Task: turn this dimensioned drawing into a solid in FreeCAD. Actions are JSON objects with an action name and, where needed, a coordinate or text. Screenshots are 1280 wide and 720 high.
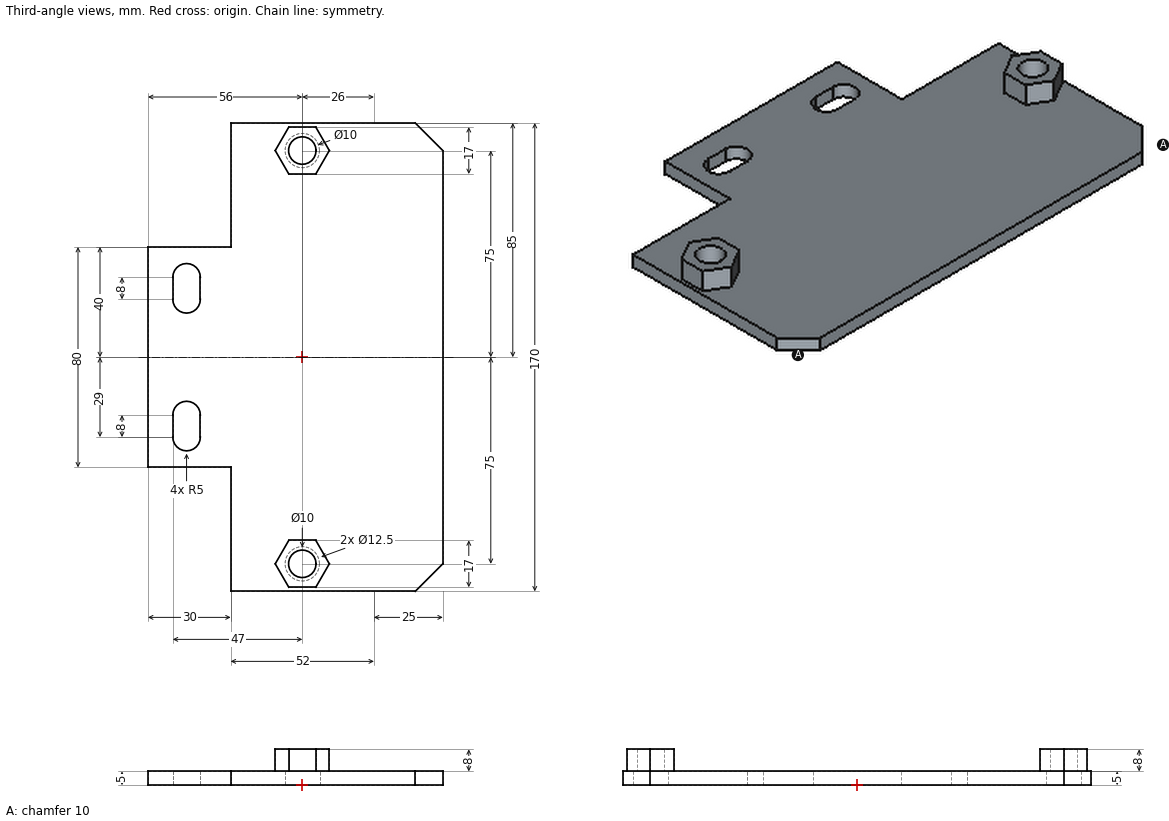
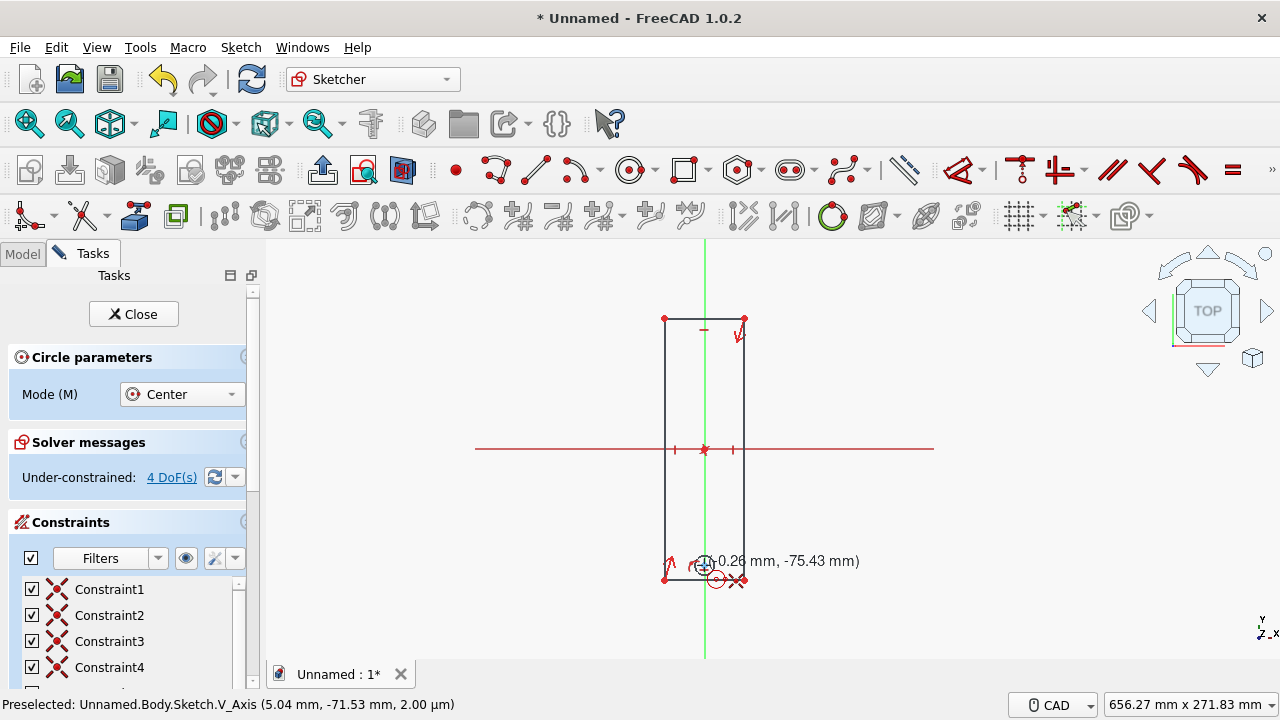
{"action": "scroll", "coordinate": [705, 333], "scroll_direction": "up", "scroll_amount": 5}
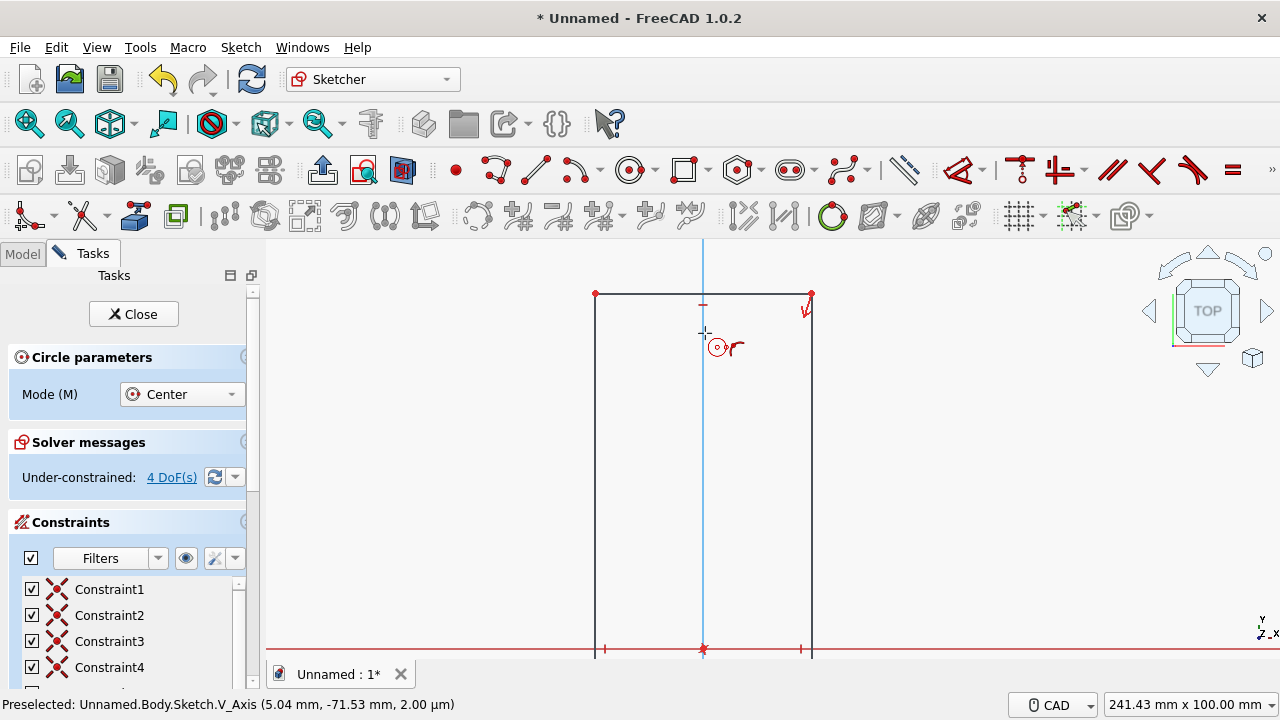
{"action": "left_click", "coordinate": [703, 334]}
{"action": "left_click", "coordinate": [722, 315]}
{"action": "key", "text": "Escape"}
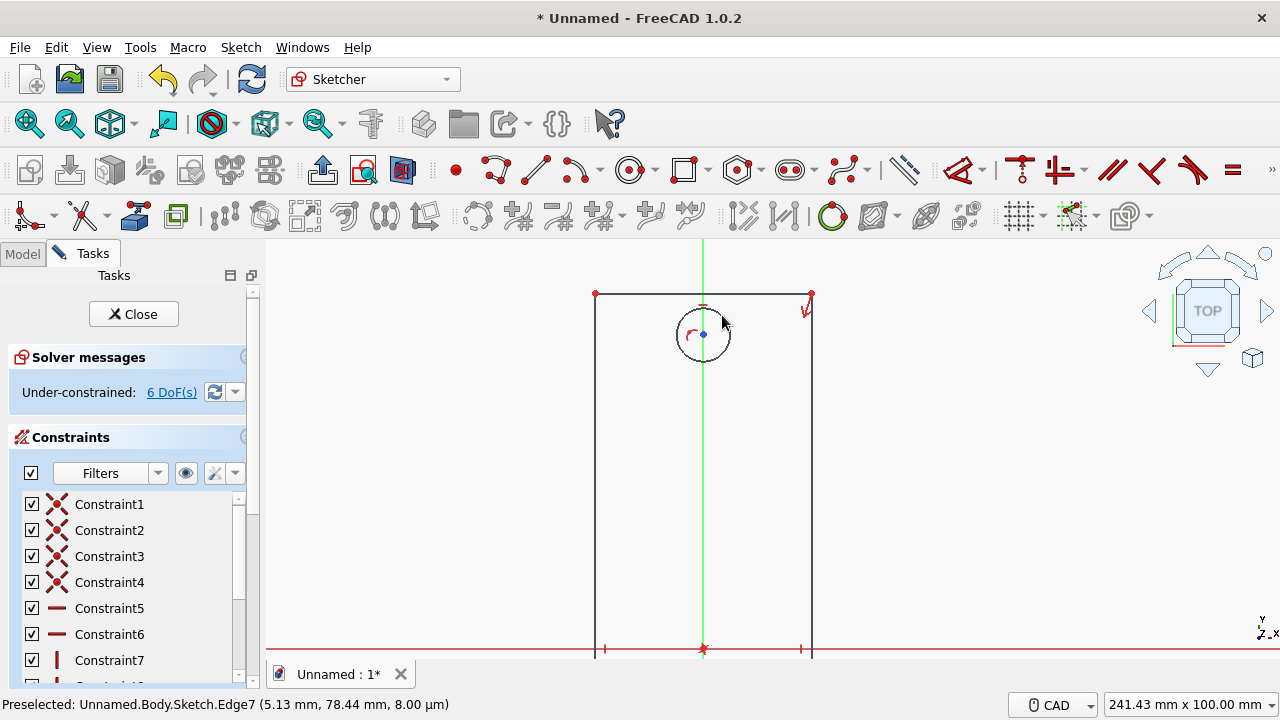
{"action": "scroll", "coordinate": [705, 333], "scroll_direction": "down", "scroll_amount": 5}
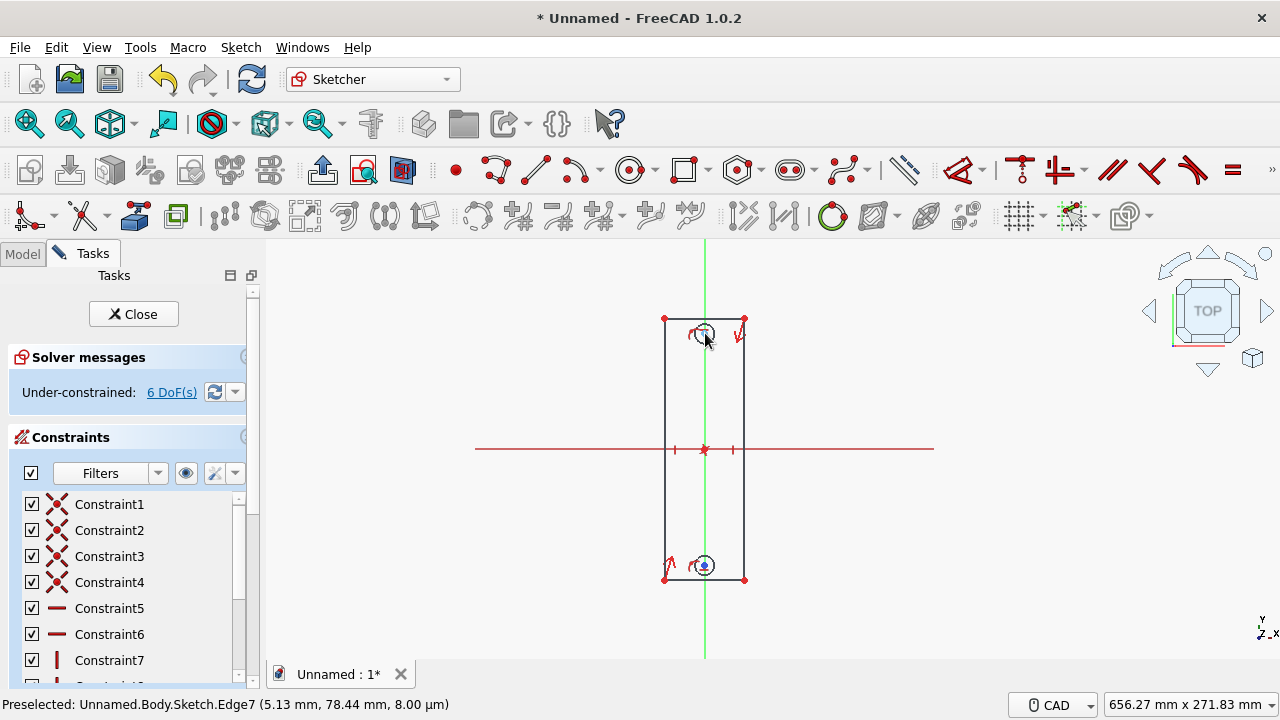
{"action": "scroll", "coordinate": [711, 559], "scroll_direction": "up", "scroll_amount": 4}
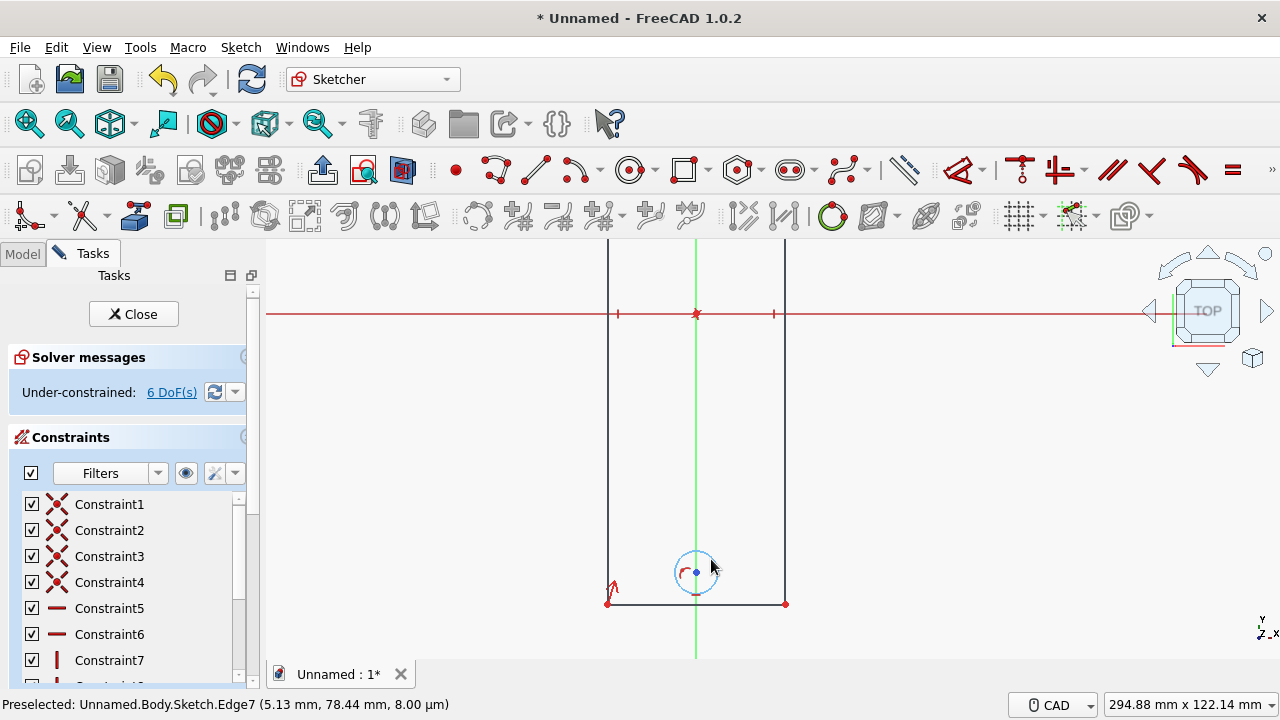
{"action": "left_click", "coordinate": [711, 557]}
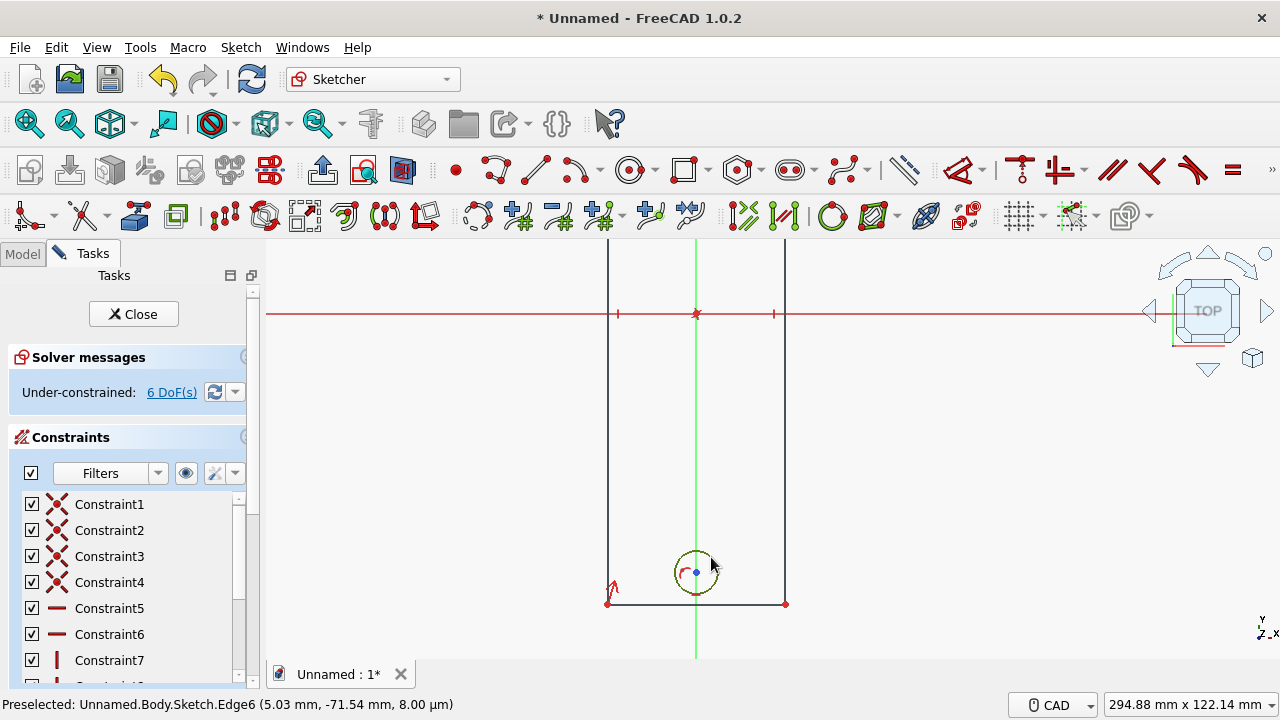
{"action": "scroll", "coordinate": [711, 559], "scroll_direction": "down", "scroll_amount": 4}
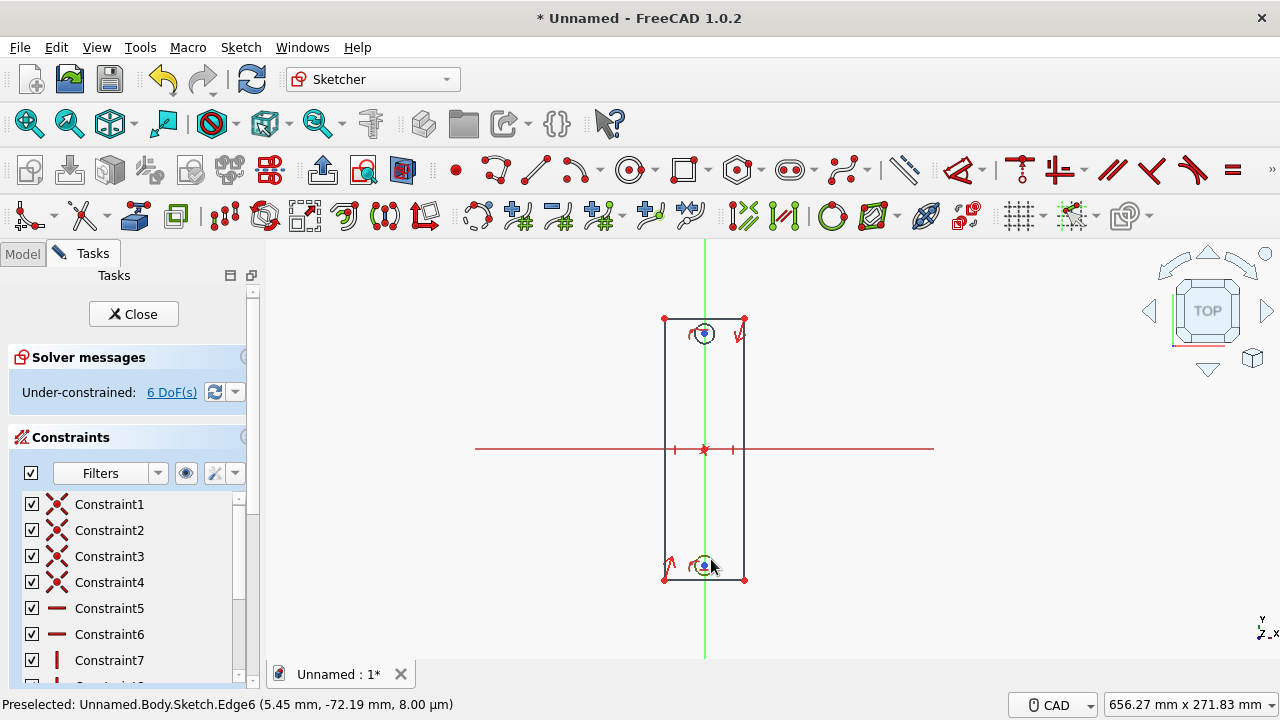
{"action": "scroll", "coordinate": [712, 327], "scroll_direction": "up", "scroll_amount": 4}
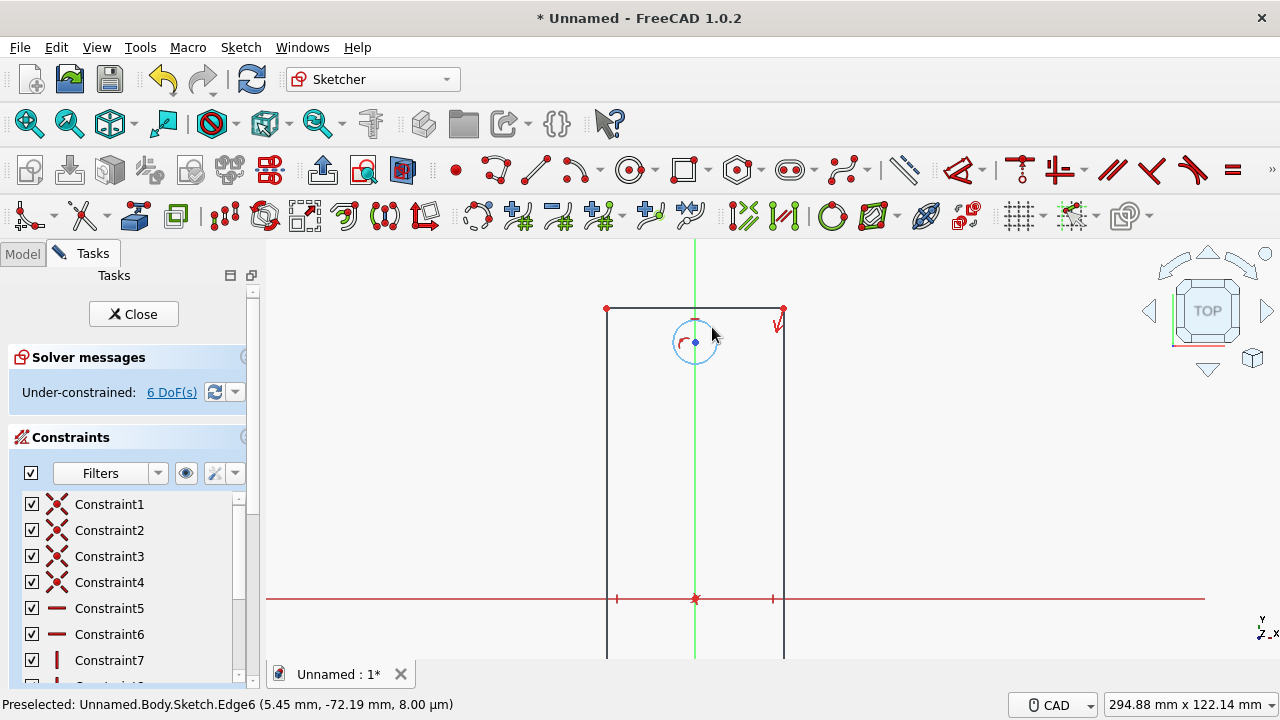
{"action": "left_click", "coordinate": [711, 327]}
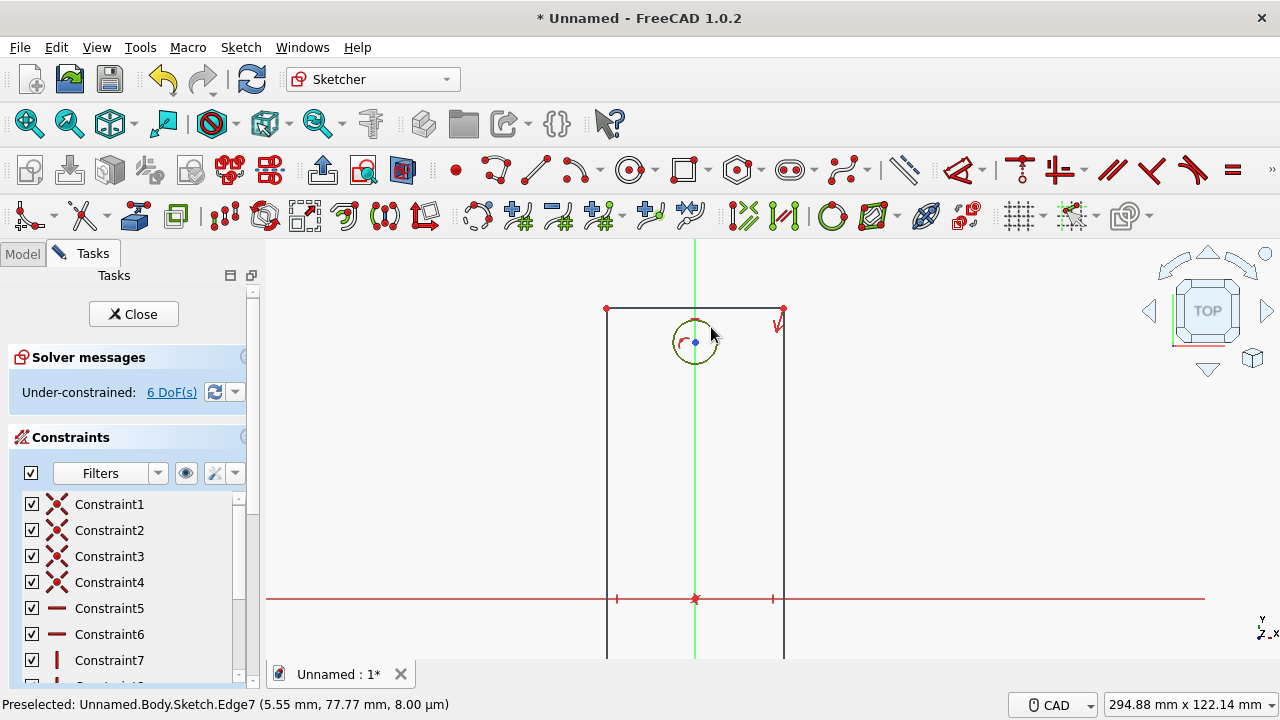
{"action": "left_click", "coordinate": [1234, 170]}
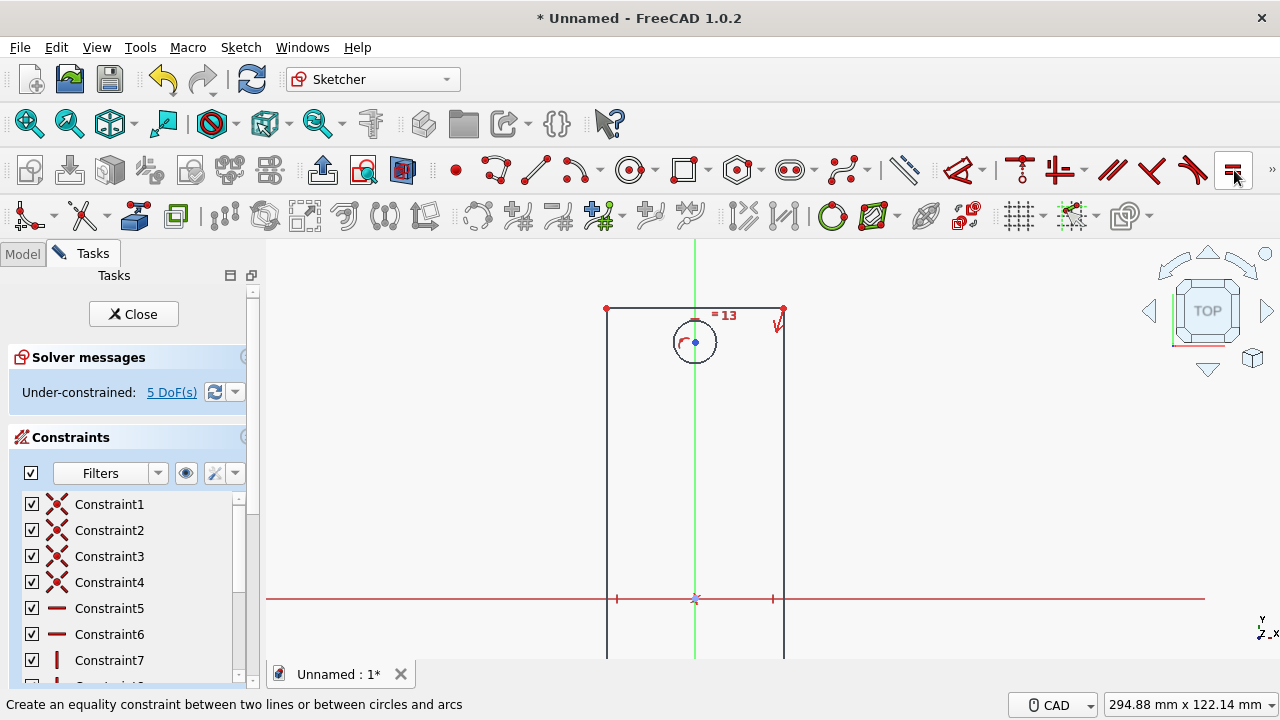
{"action": "left_click", "coordinate": [958, 170]}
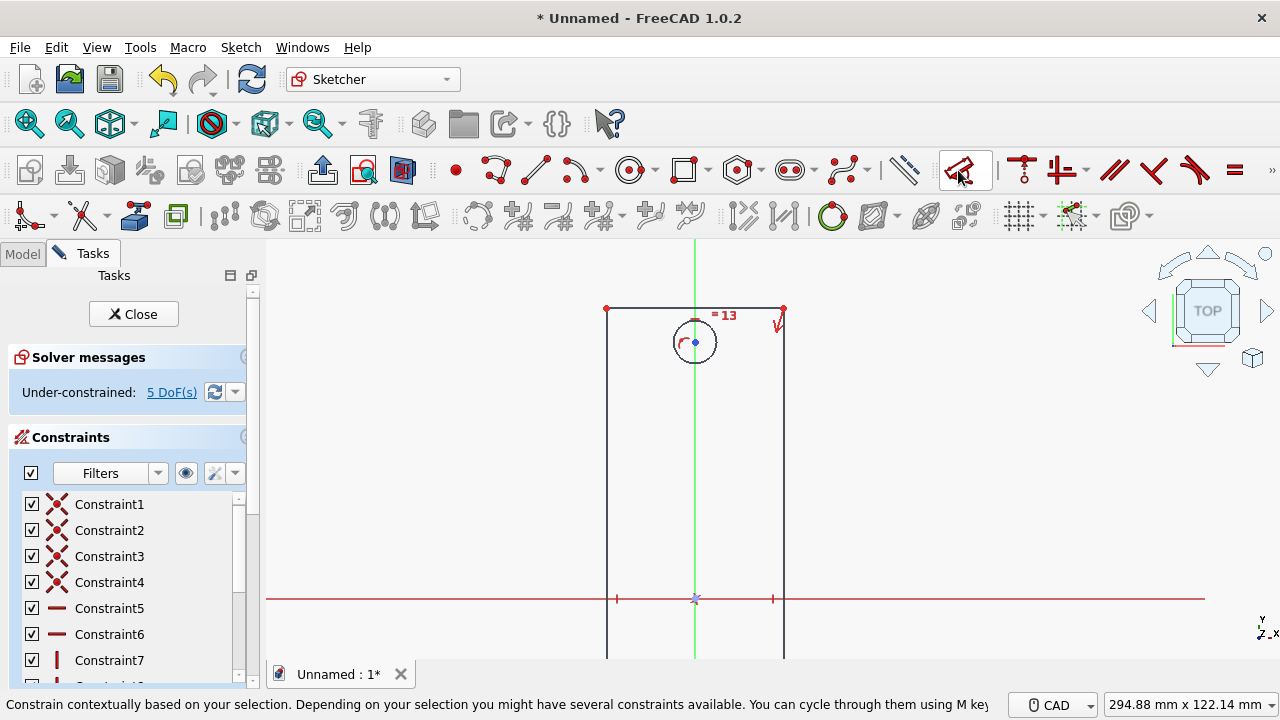
{"action": "scroll", "coordinate": [712, 327], "scroll_direction": "down", "scroll_amount": 4}